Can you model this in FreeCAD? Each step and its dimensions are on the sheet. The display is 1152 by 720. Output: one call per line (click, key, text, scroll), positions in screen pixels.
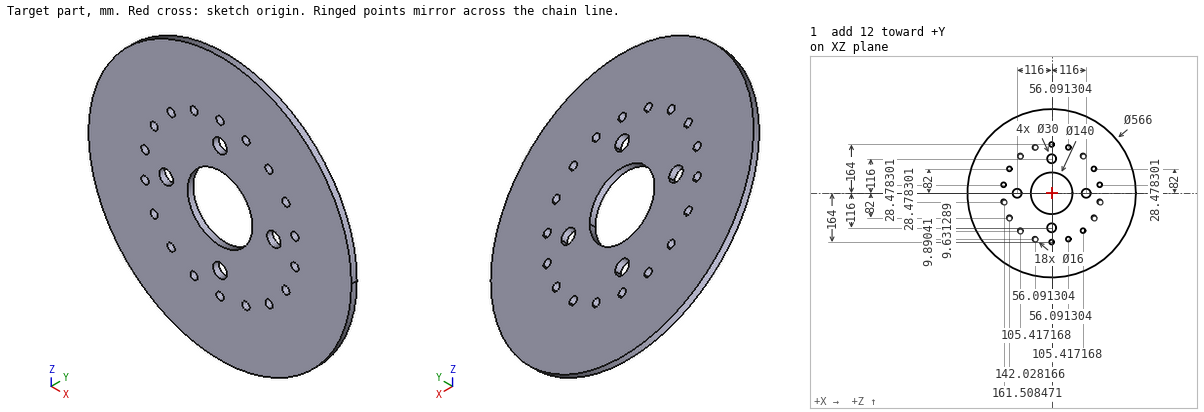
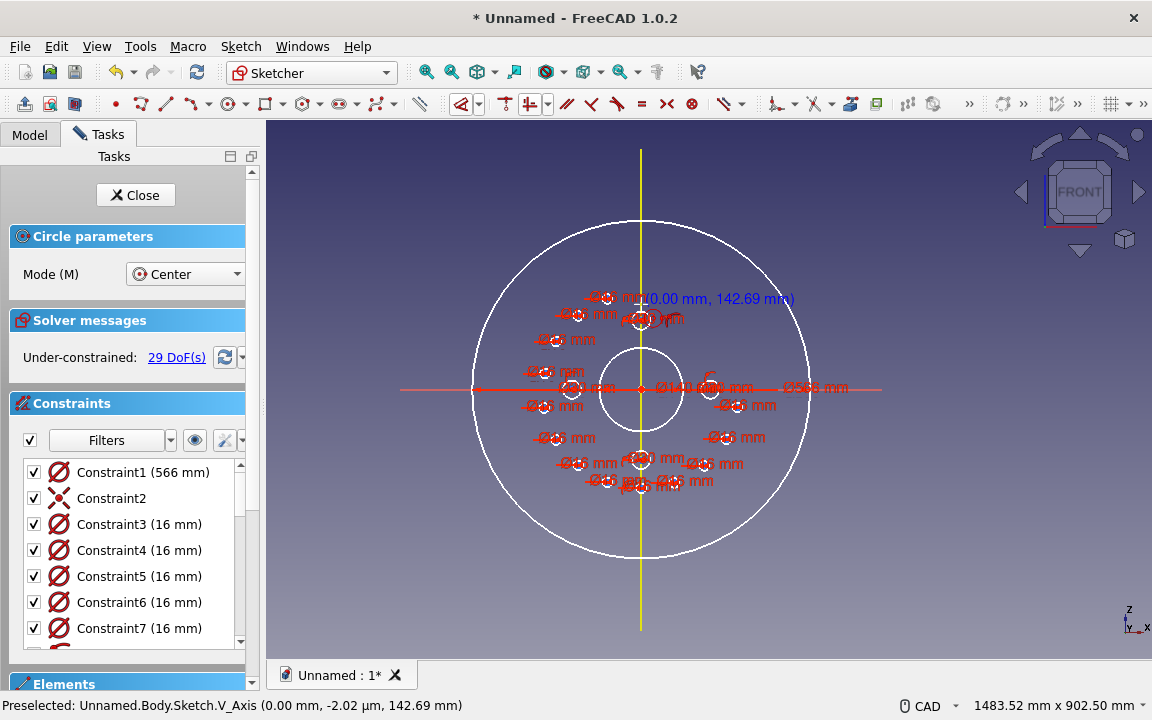
click(641, 292)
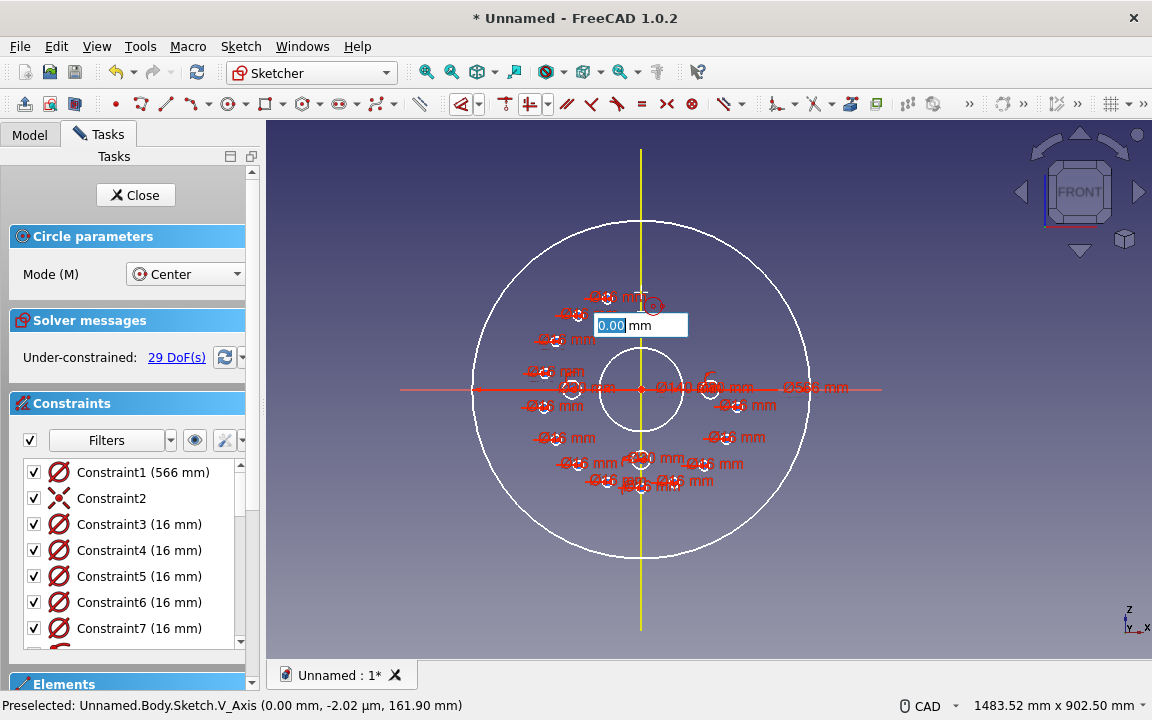
scroll(646, 290, up, 7)
move(643, 289)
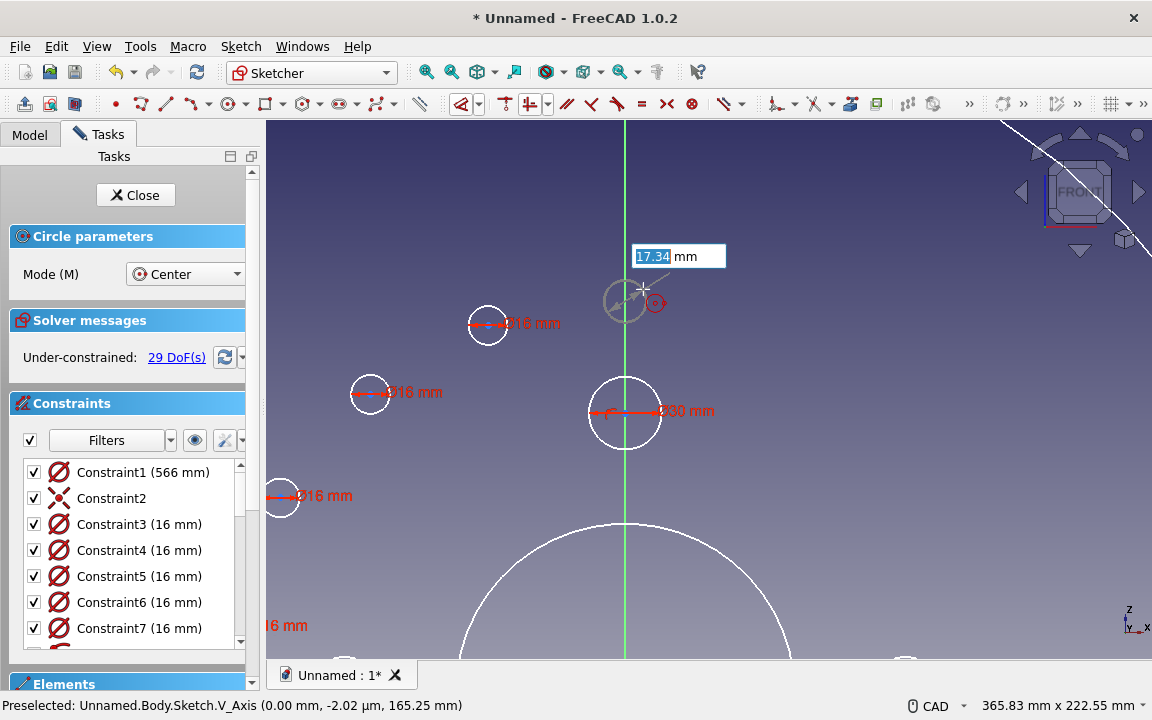
text(16)
key(Return)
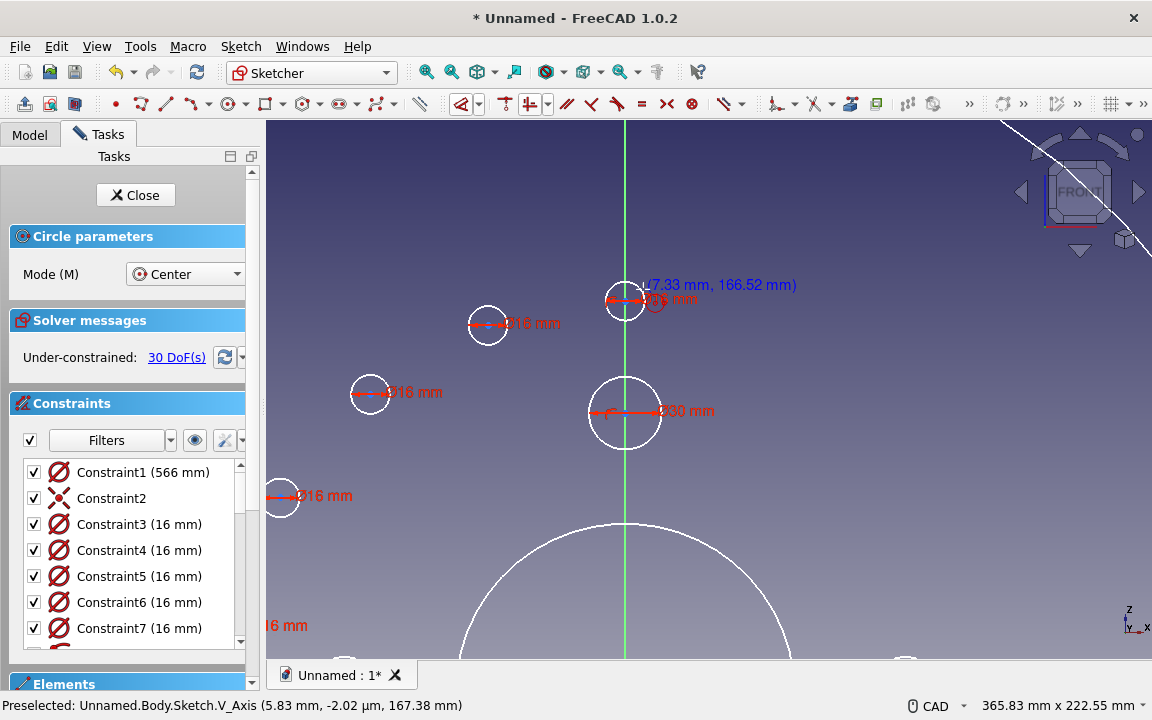
scroll(645, 290, down, 7)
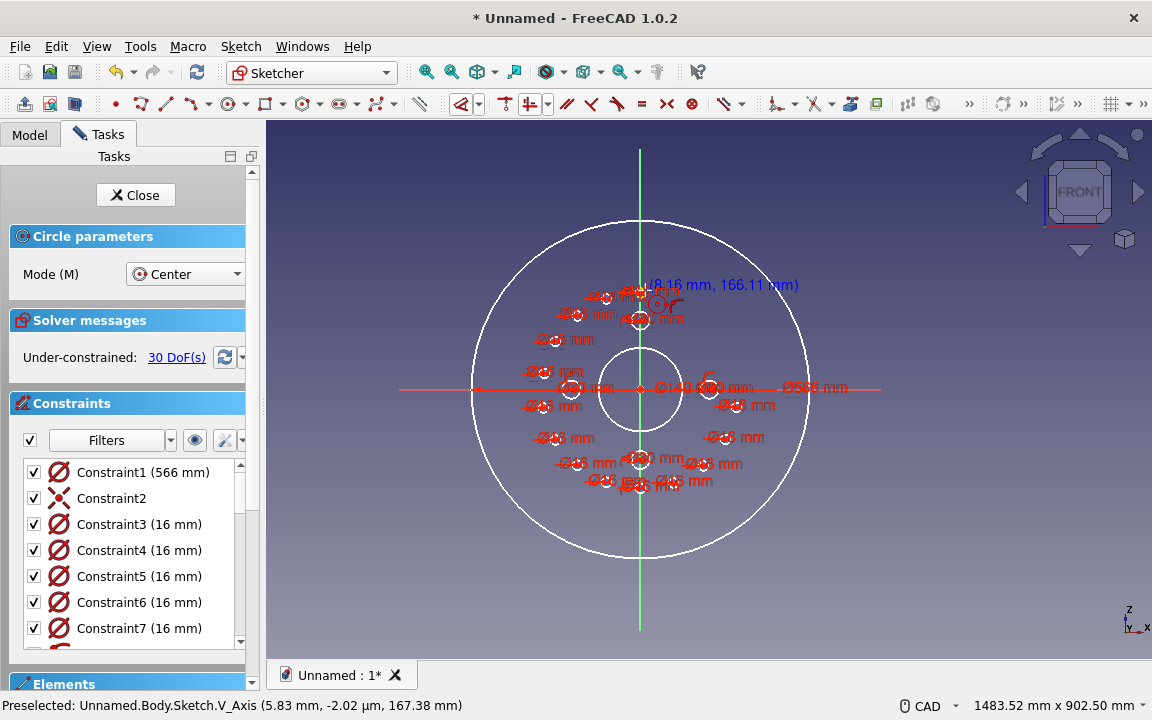
click(674, 298)
move(677, 294)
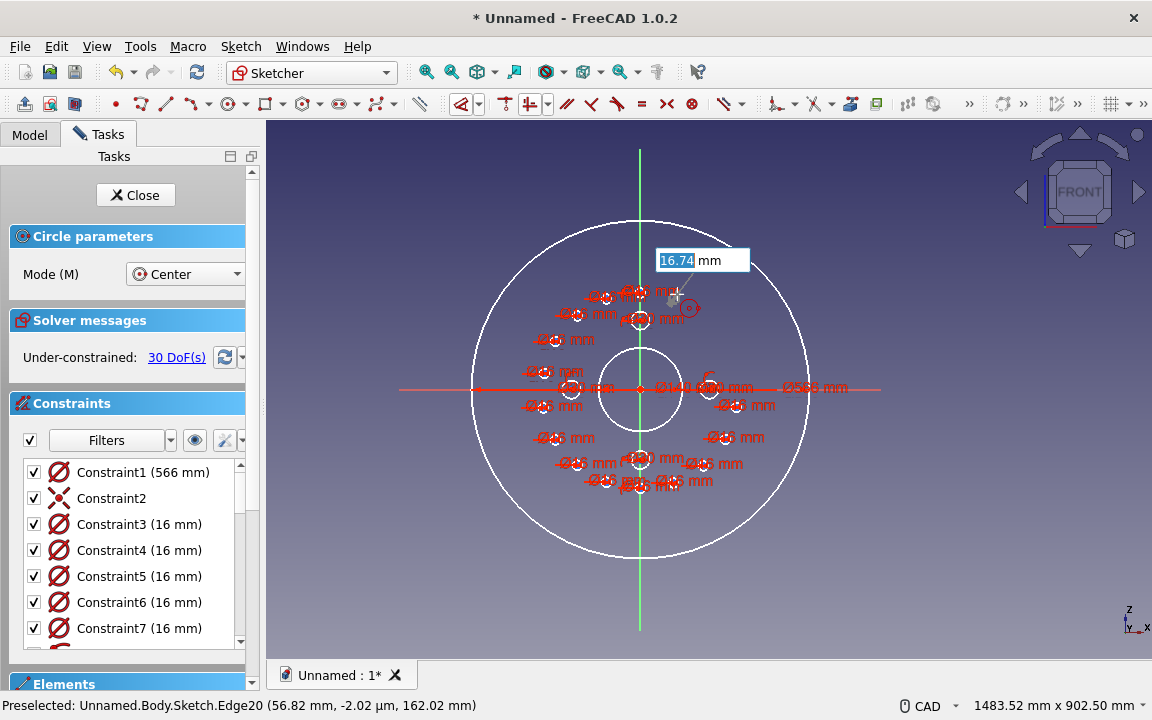
text(16)
key(Return)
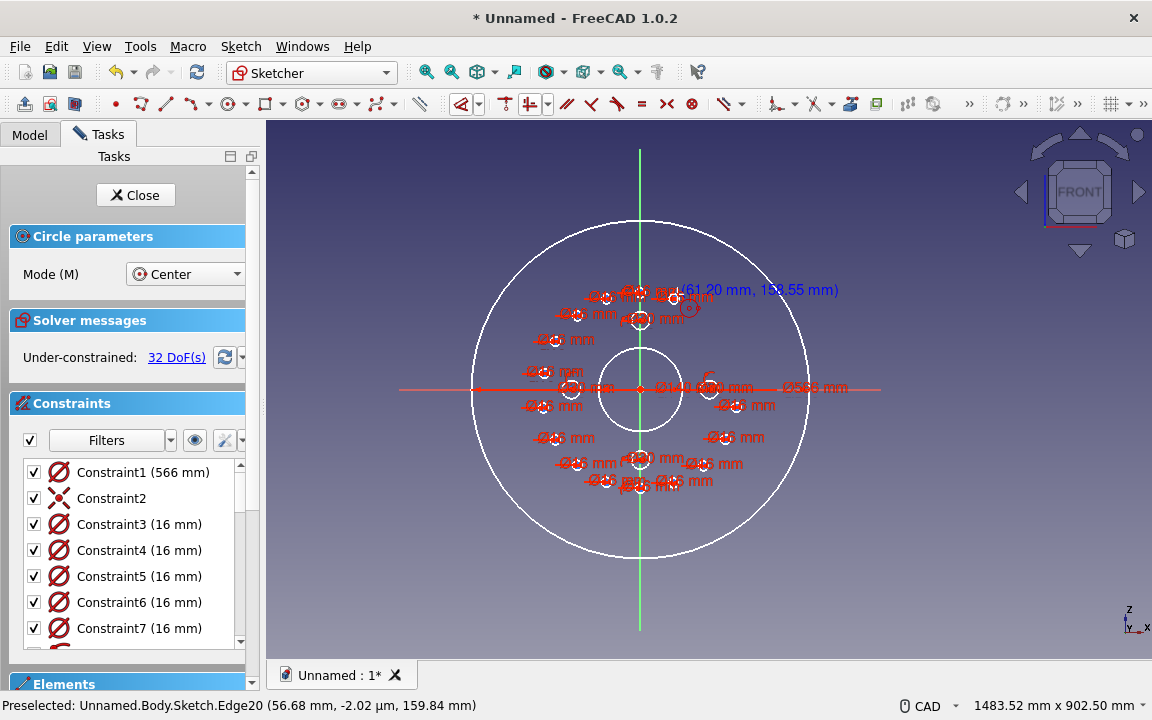
scroll(737, 373, up, 8)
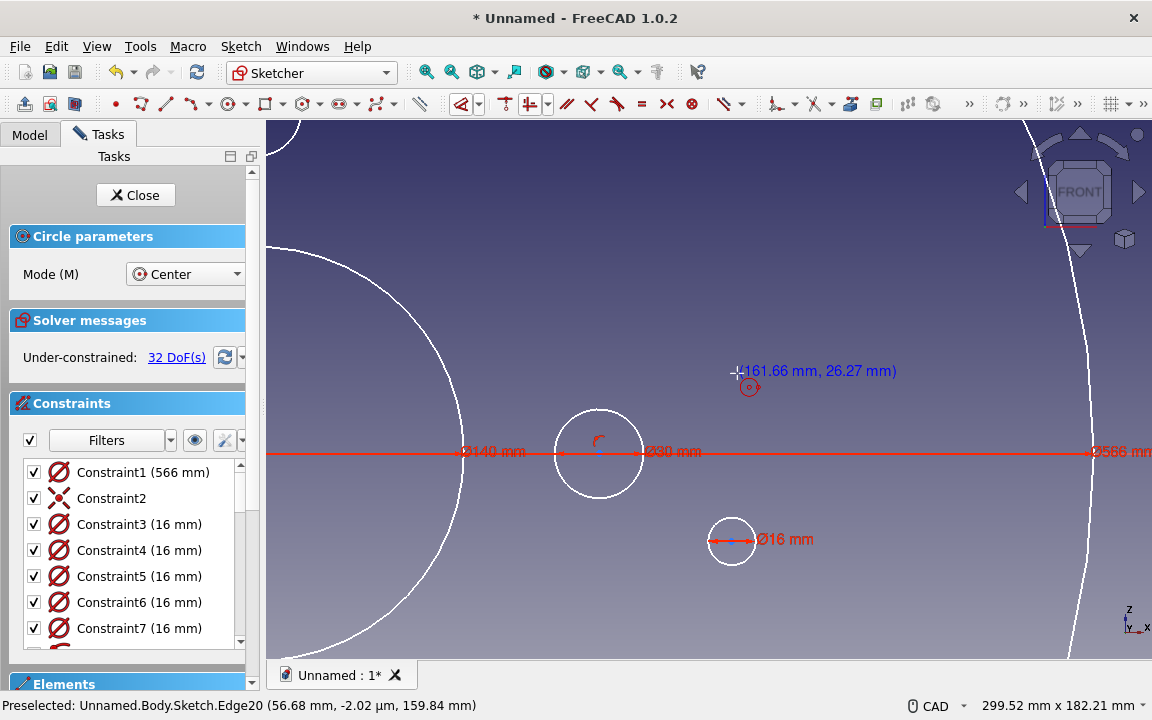
scroll(738, 373, down, 8)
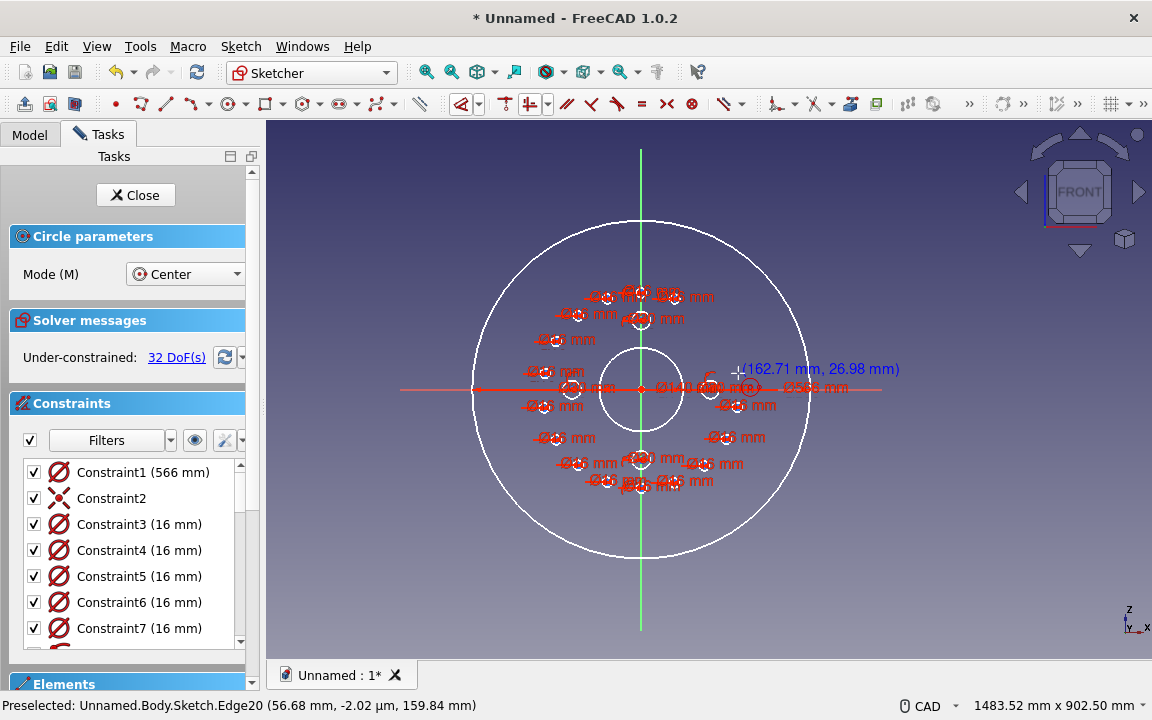
click(738, 373)
move(741, 369)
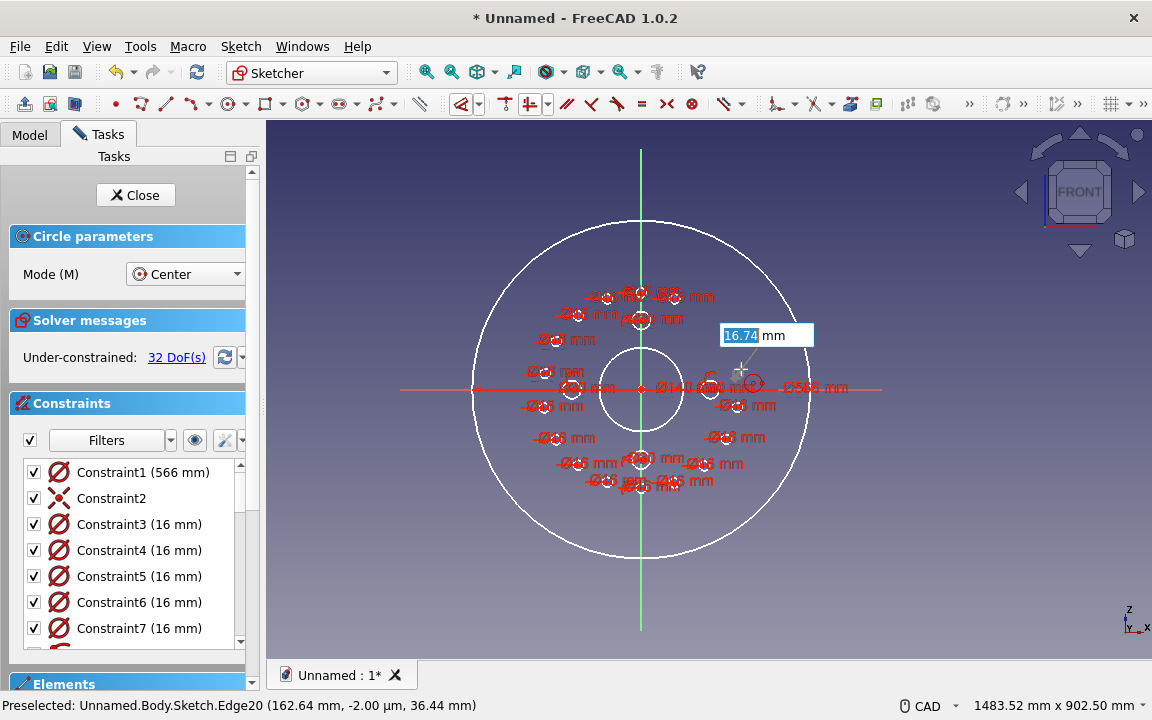
text(16)
key(Return)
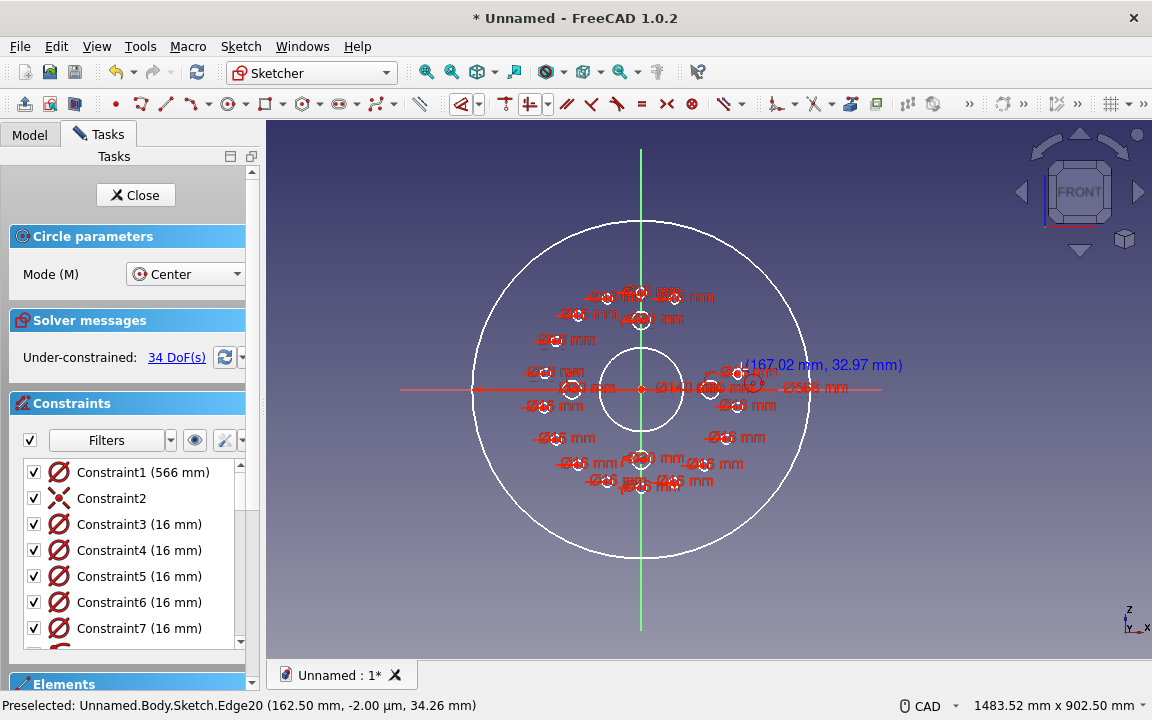
scroll(726, 341, up, 8)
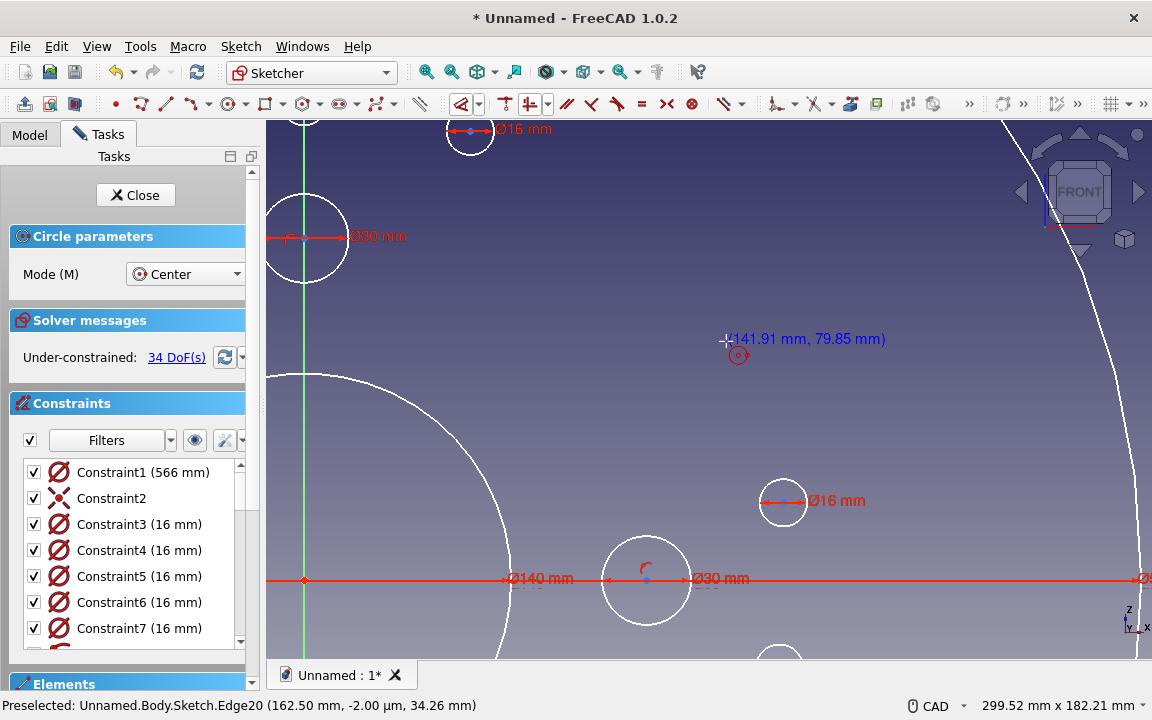
scroll(726, 341, down, 8)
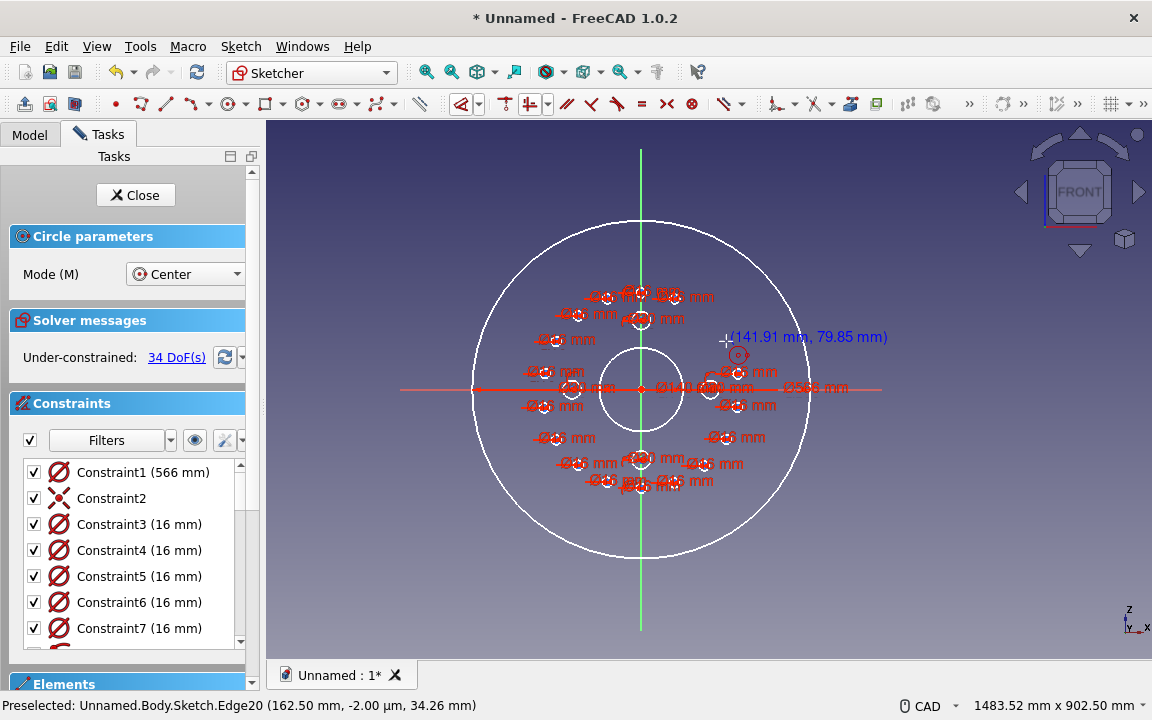
click(726, 341)
move(729, 337)